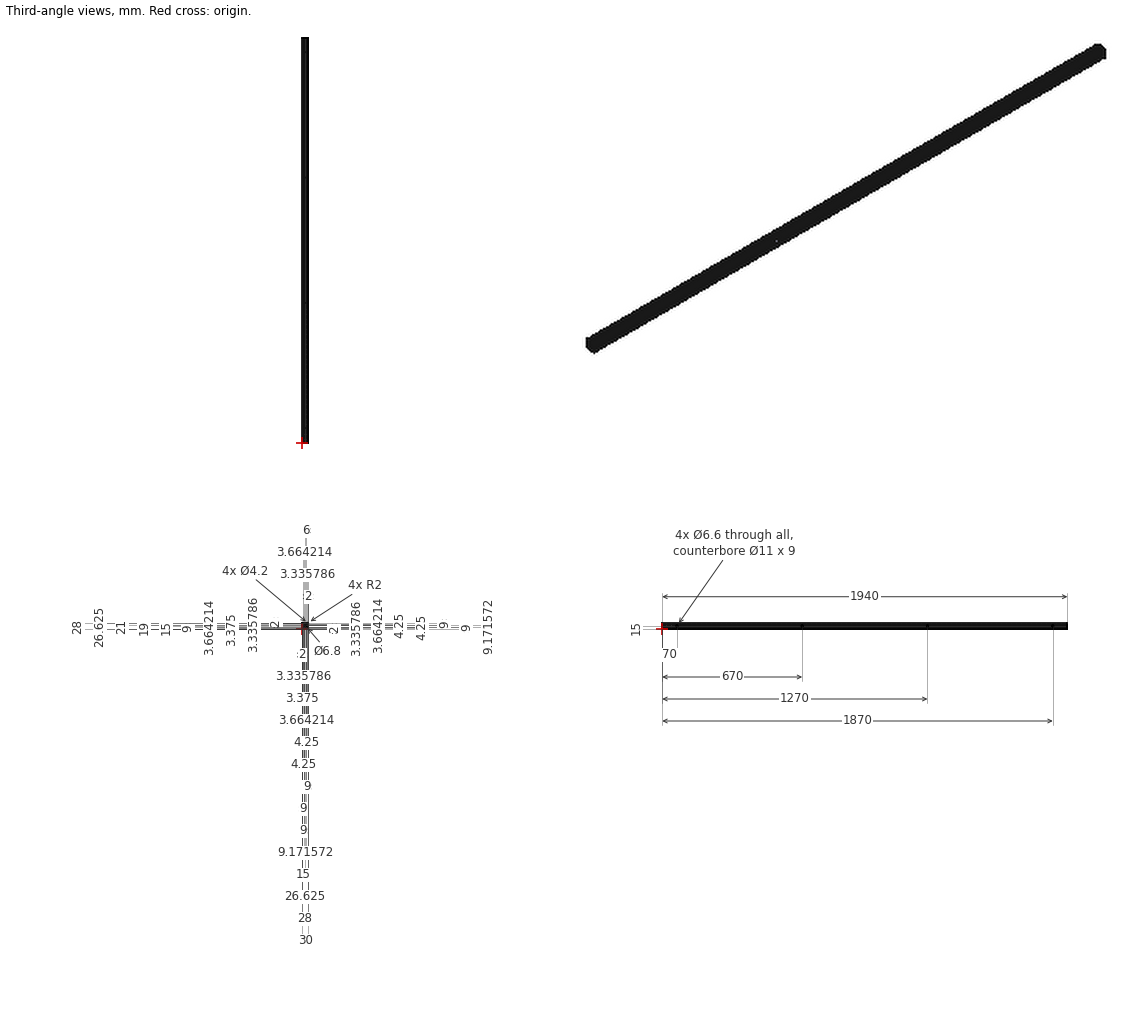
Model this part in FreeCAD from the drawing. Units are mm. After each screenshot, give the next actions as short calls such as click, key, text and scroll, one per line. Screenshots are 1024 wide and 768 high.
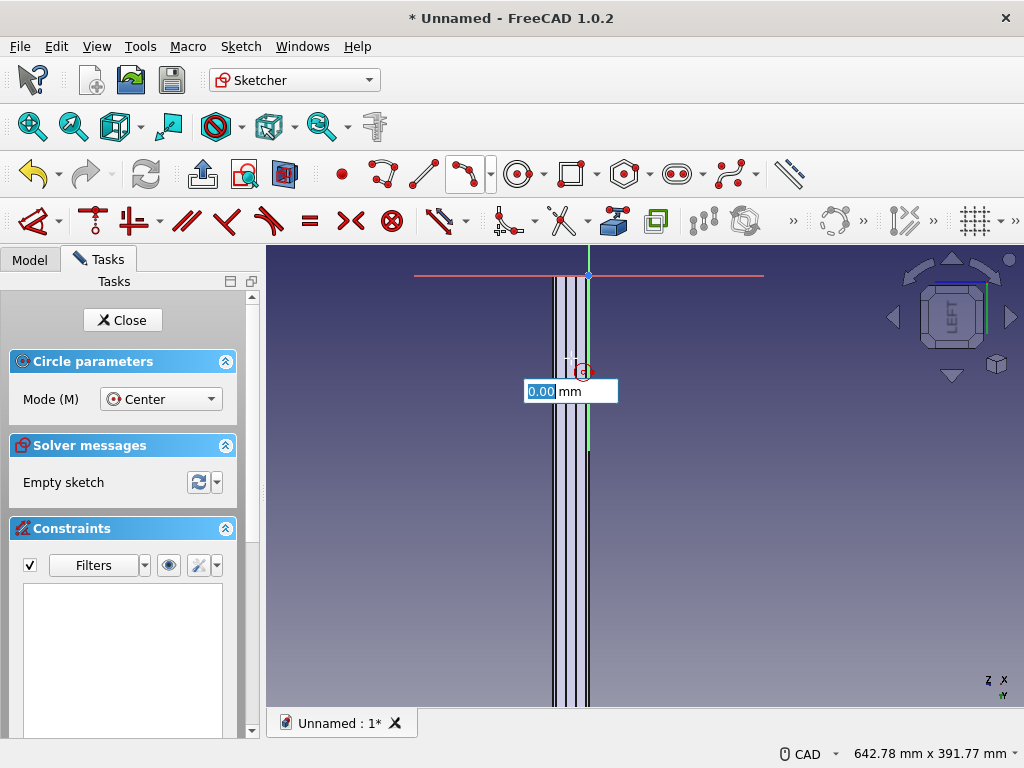
scroll(574, 356, up, 8)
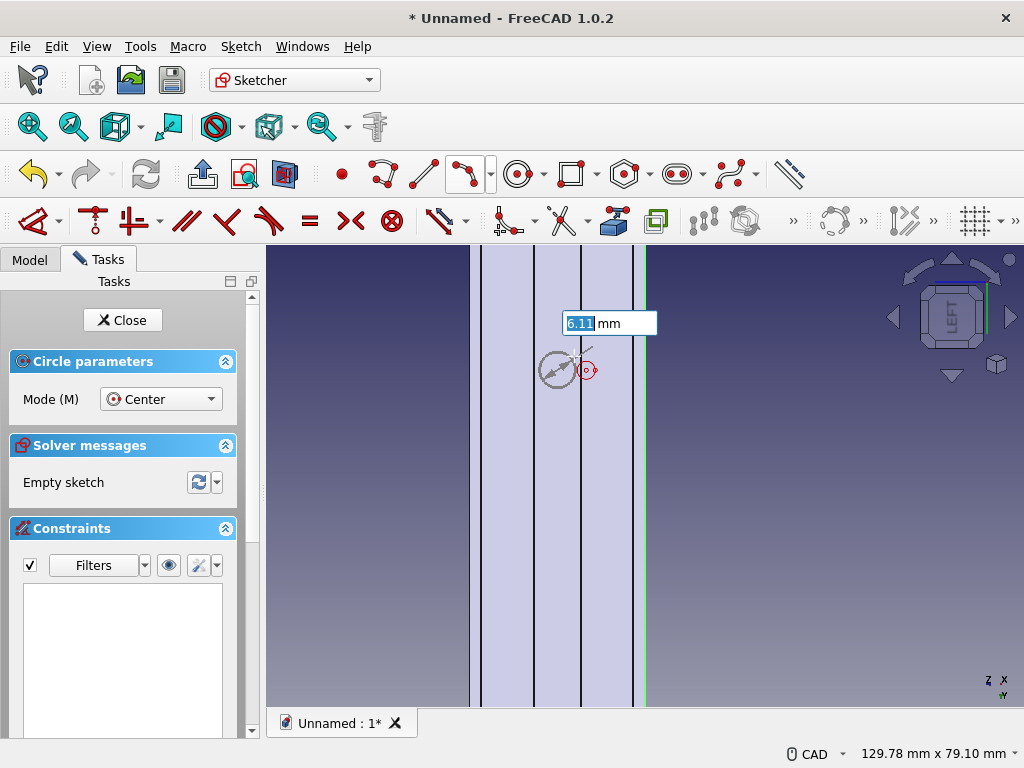
click(571, 354)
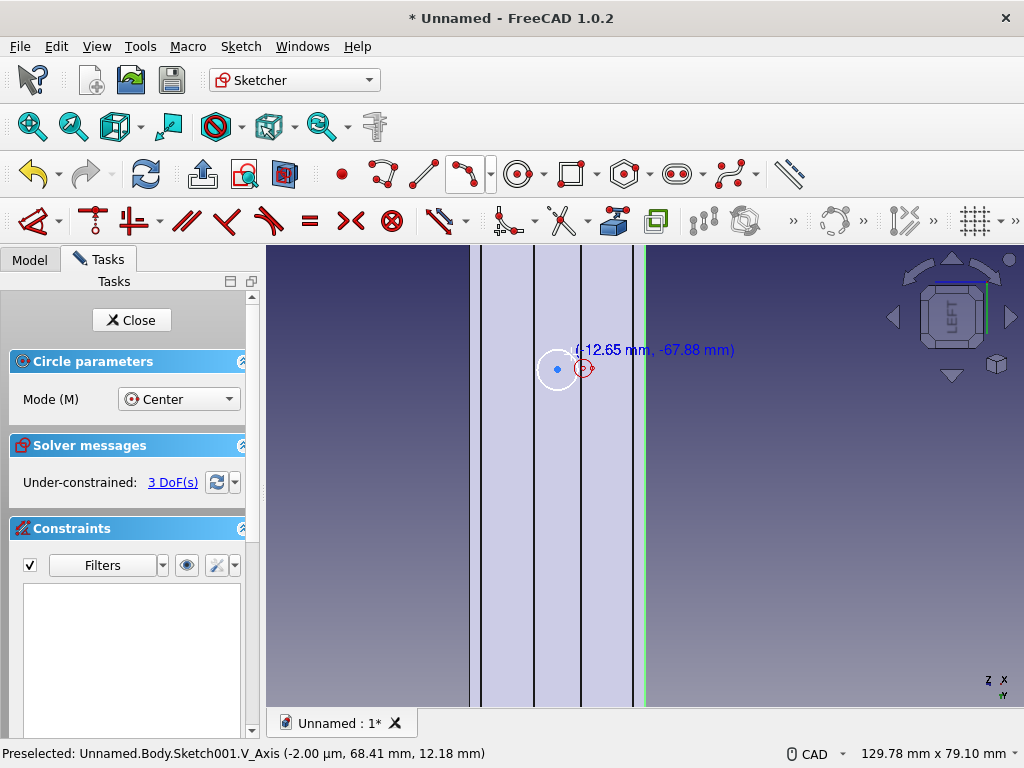
scroll(576, 337, down, 18)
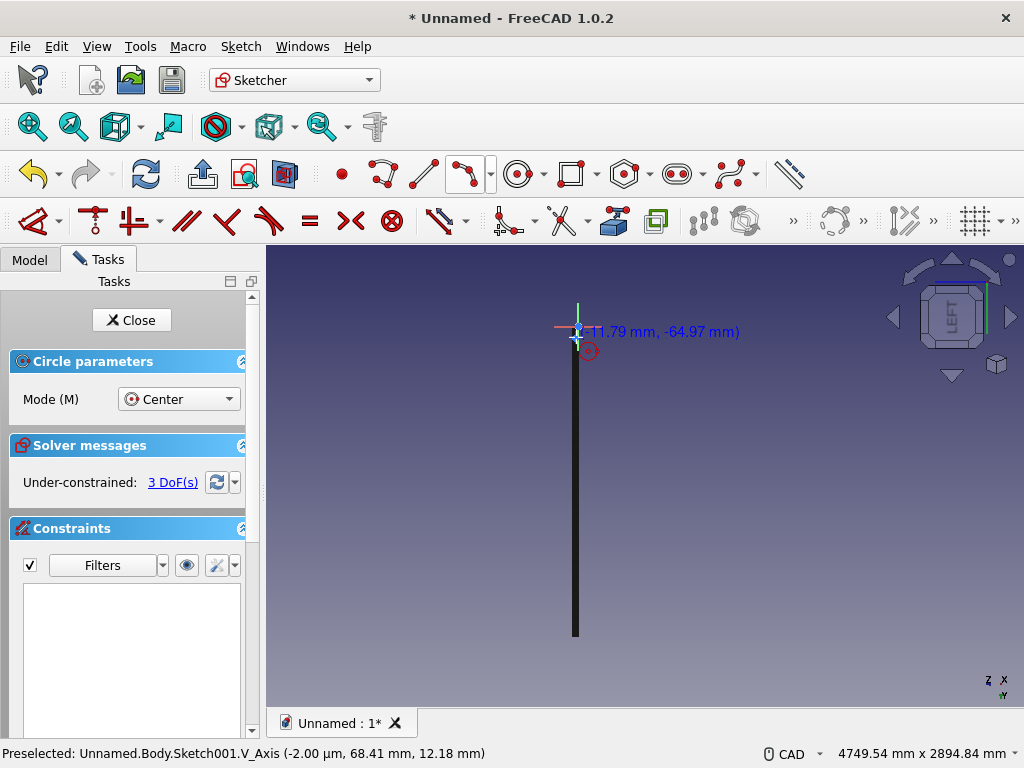
scroll(576, 625, up, 19)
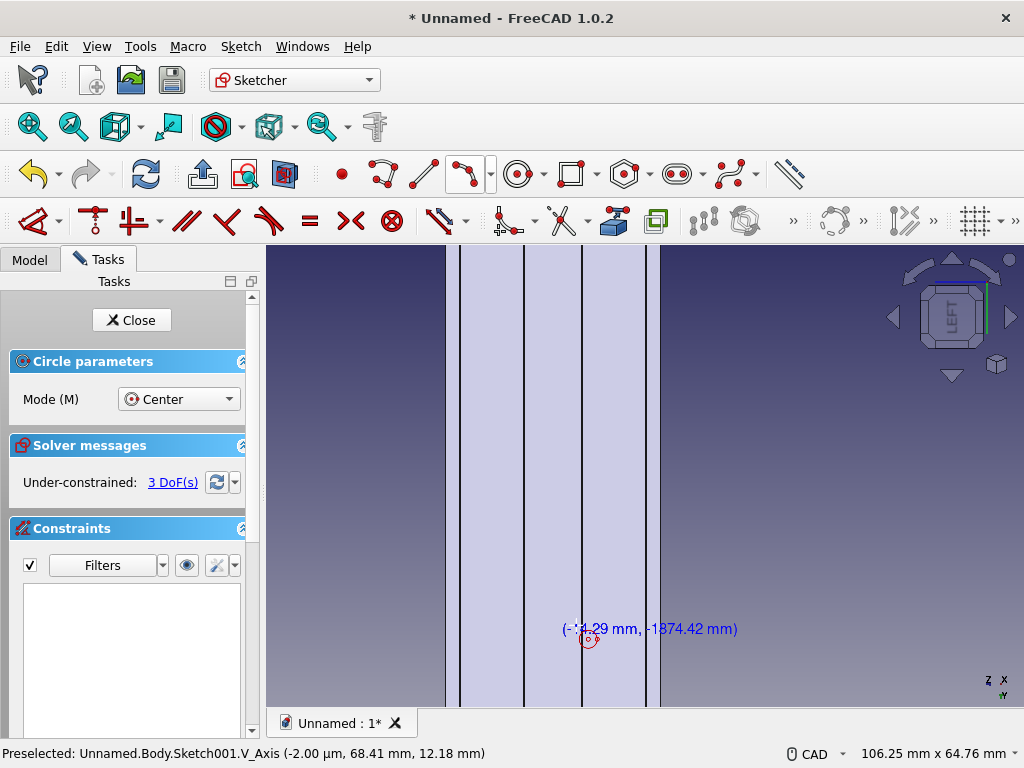
scroll(576, 476, down, 15)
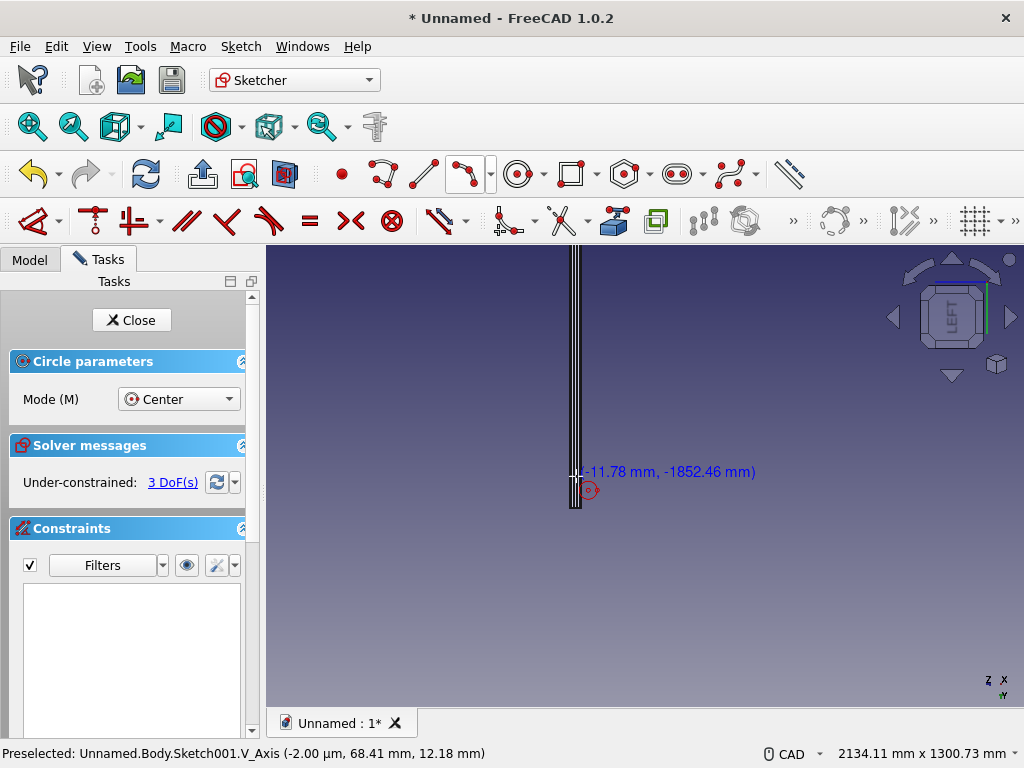
scroll(576, 665, down, 5)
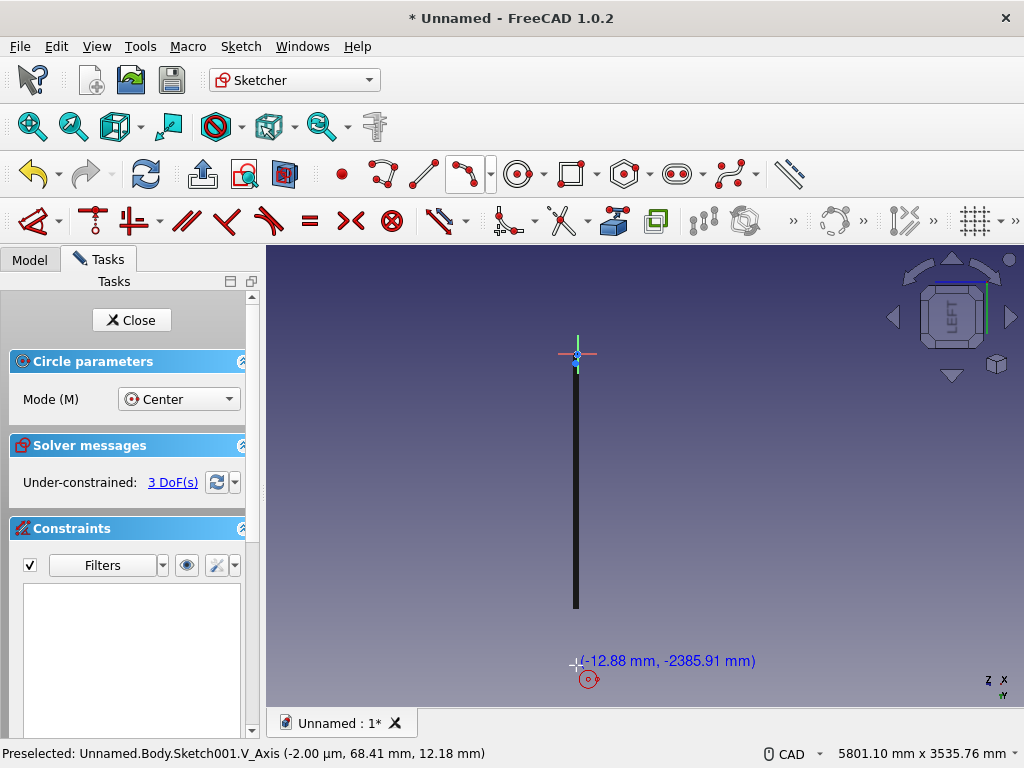
scroll(576, 599, up, 11)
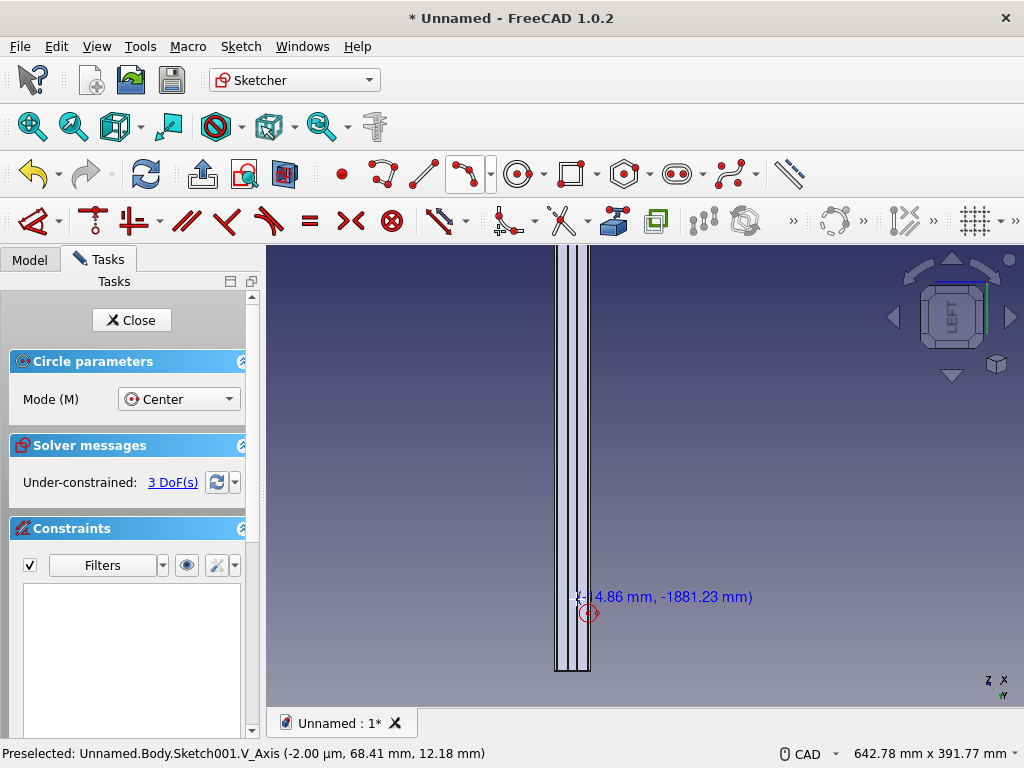
click(573, 589)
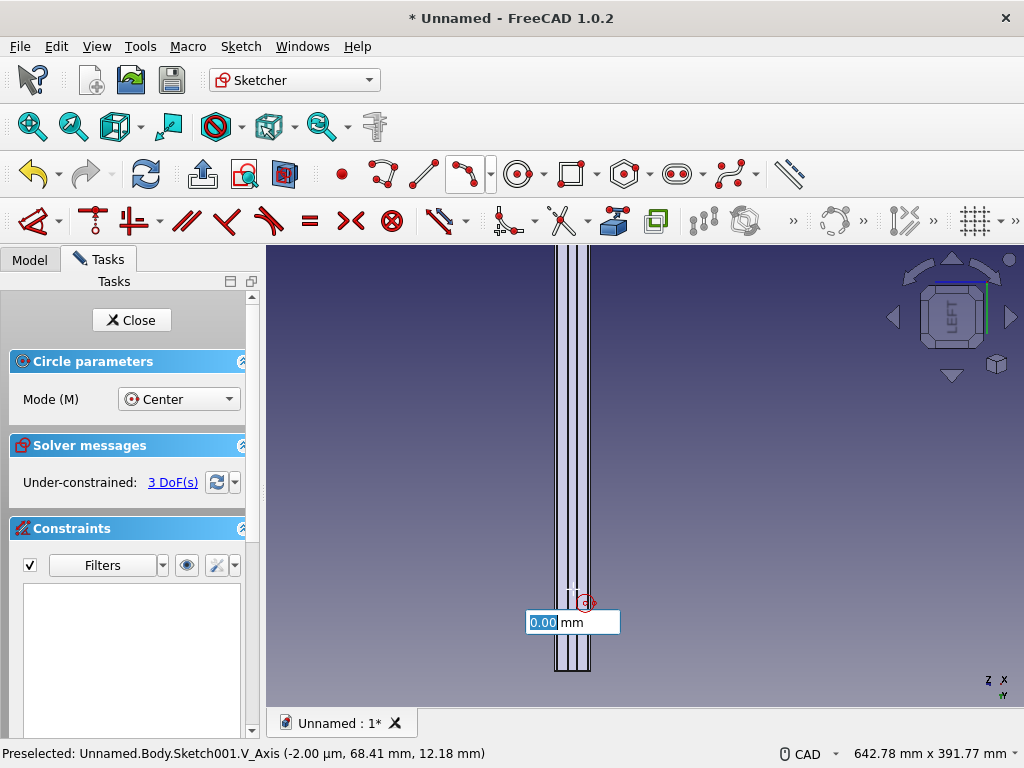
scroll(575, 586, up, 8)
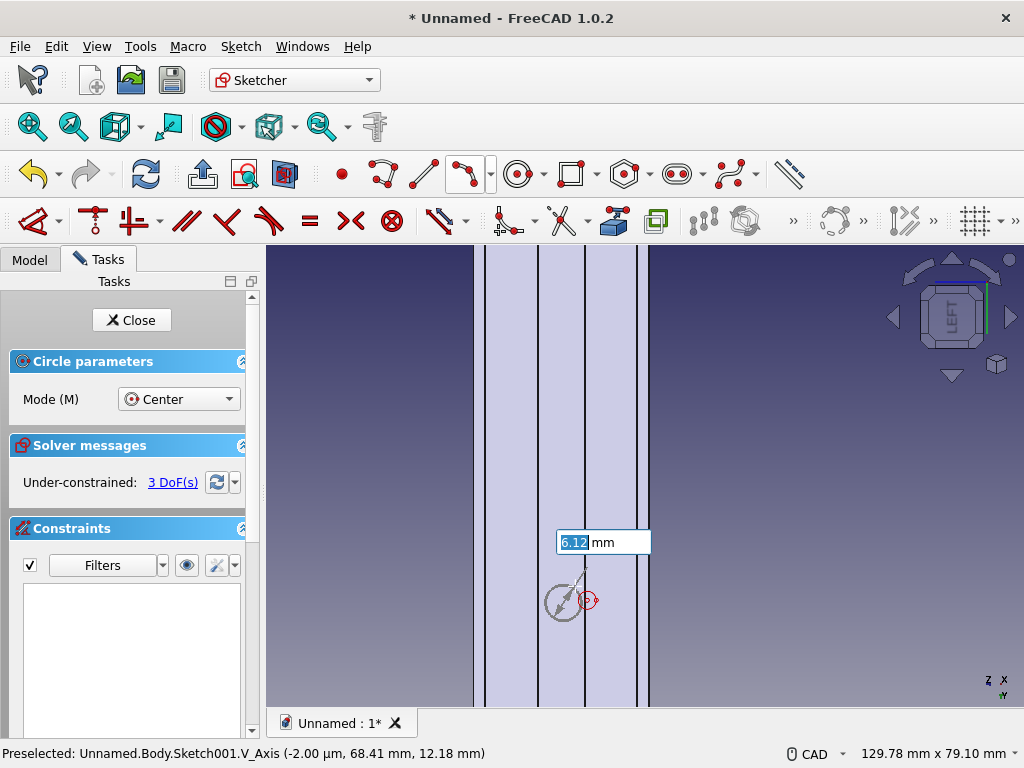
click(575, 582)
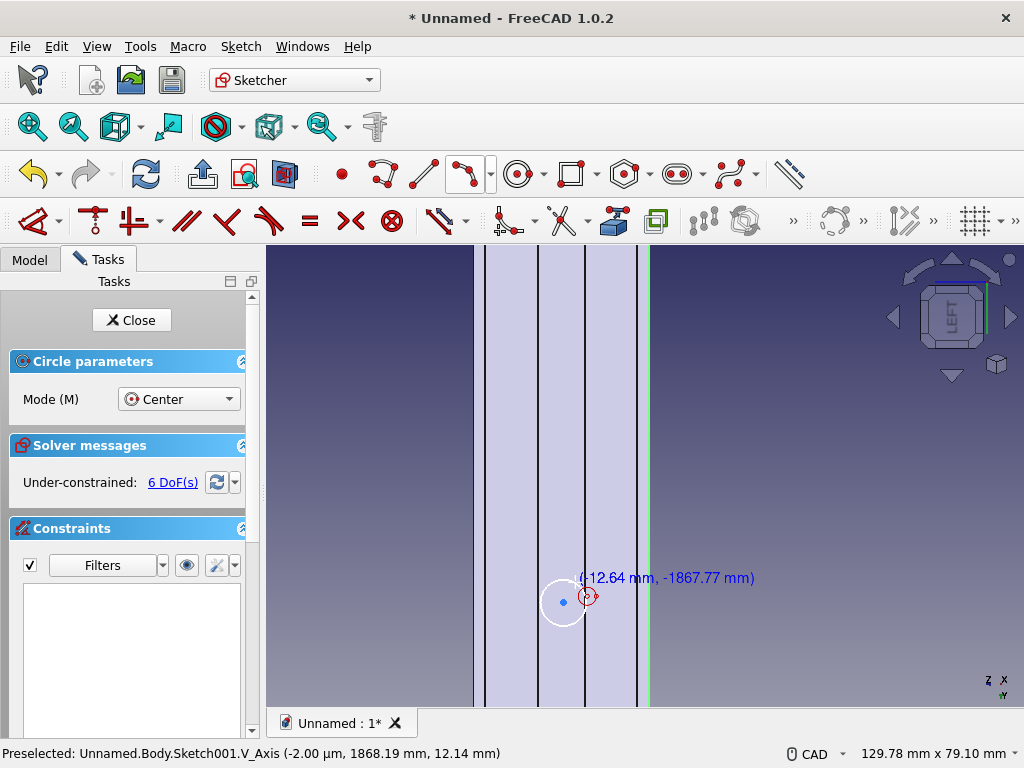
scroll(576, 626, down, 18)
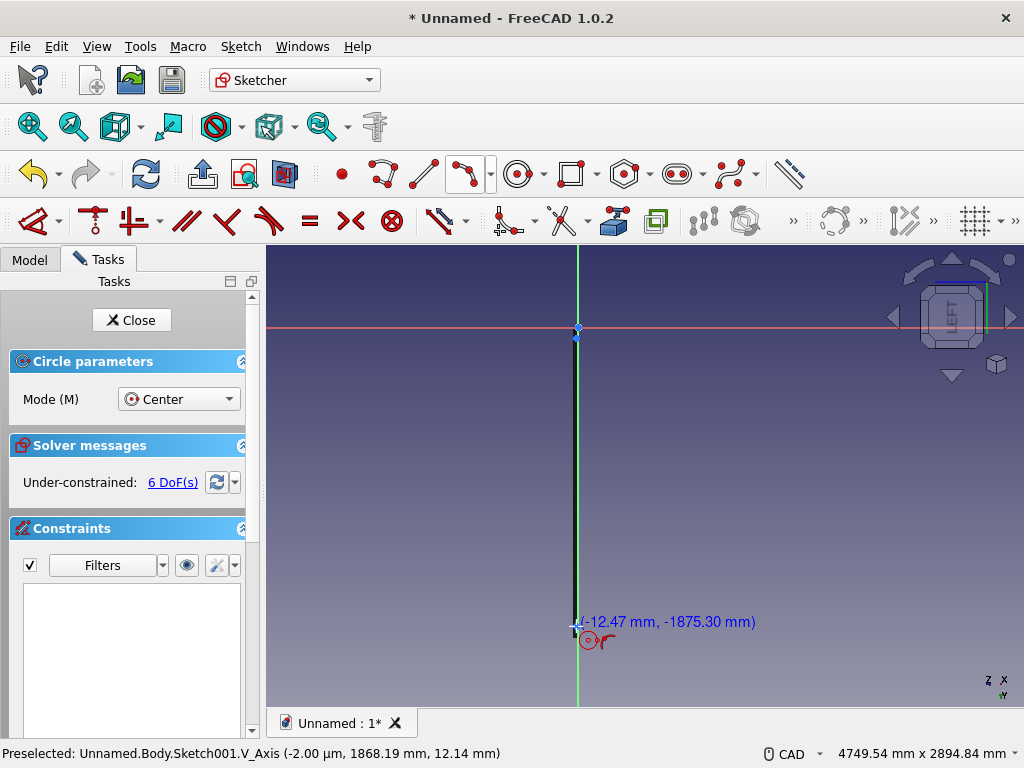
scroll(576, 530, up, 19)